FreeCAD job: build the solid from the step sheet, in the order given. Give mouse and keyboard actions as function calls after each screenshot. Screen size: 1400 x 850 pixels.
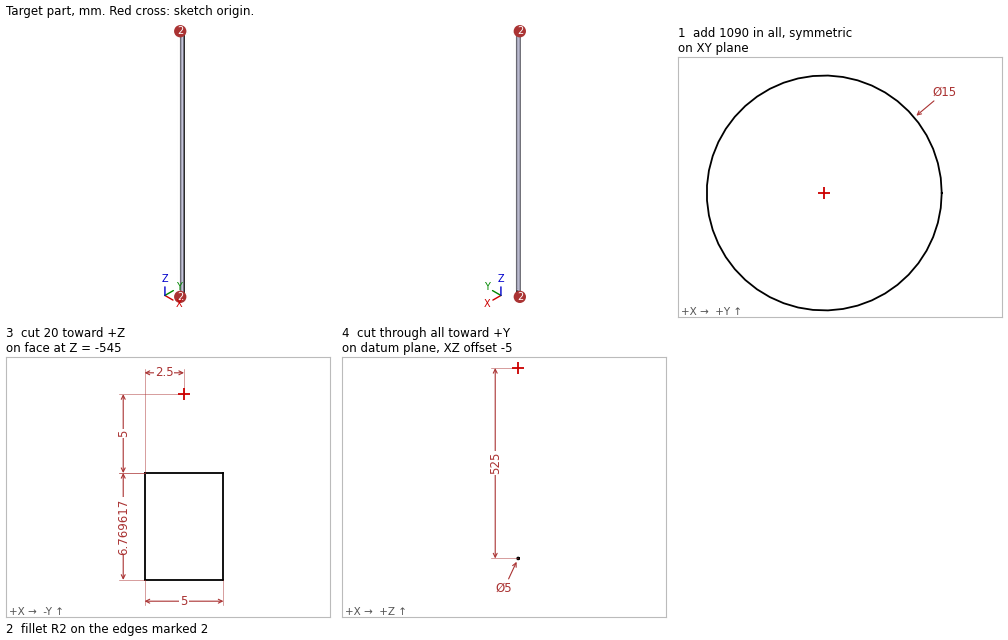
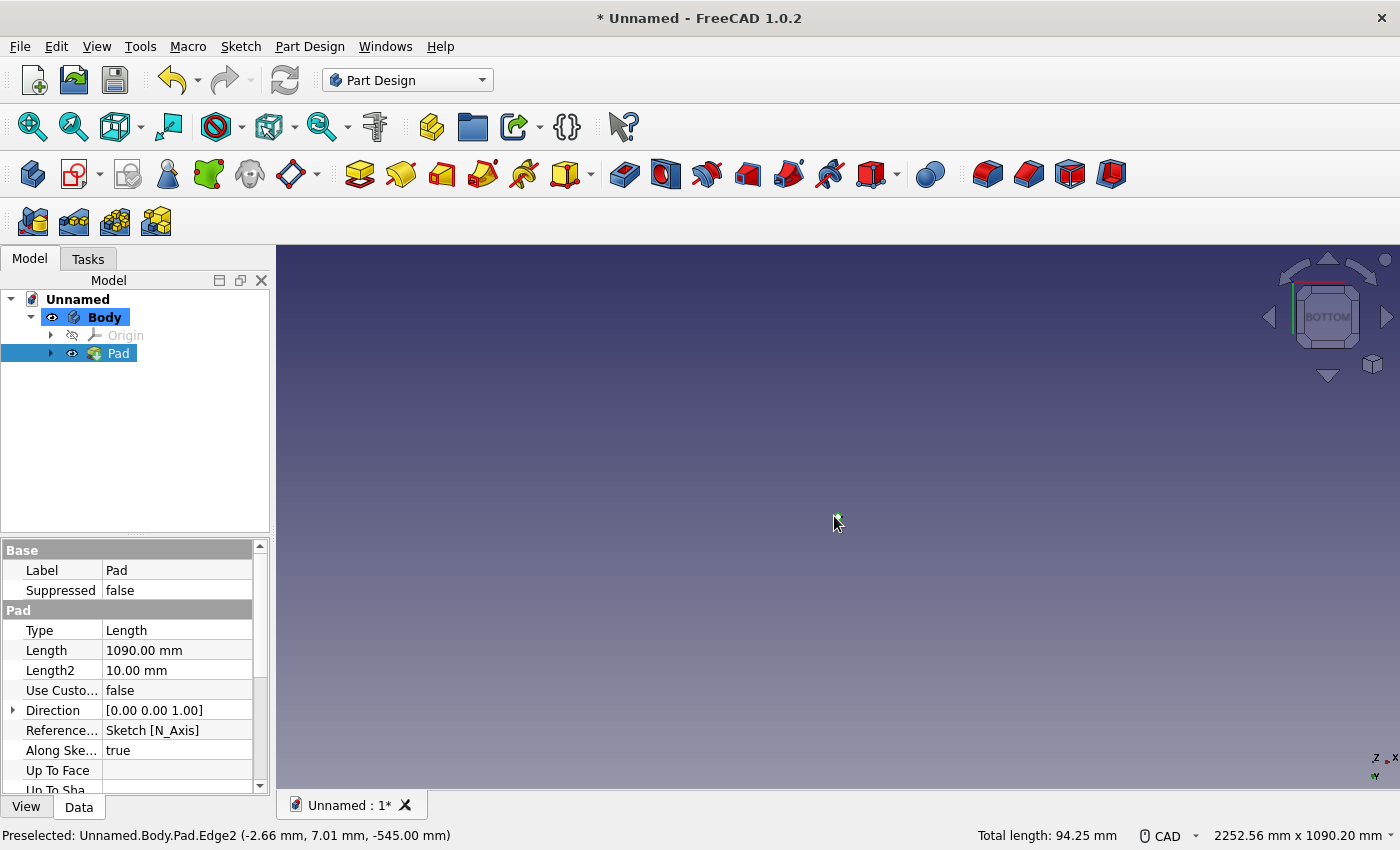
click(988, 174)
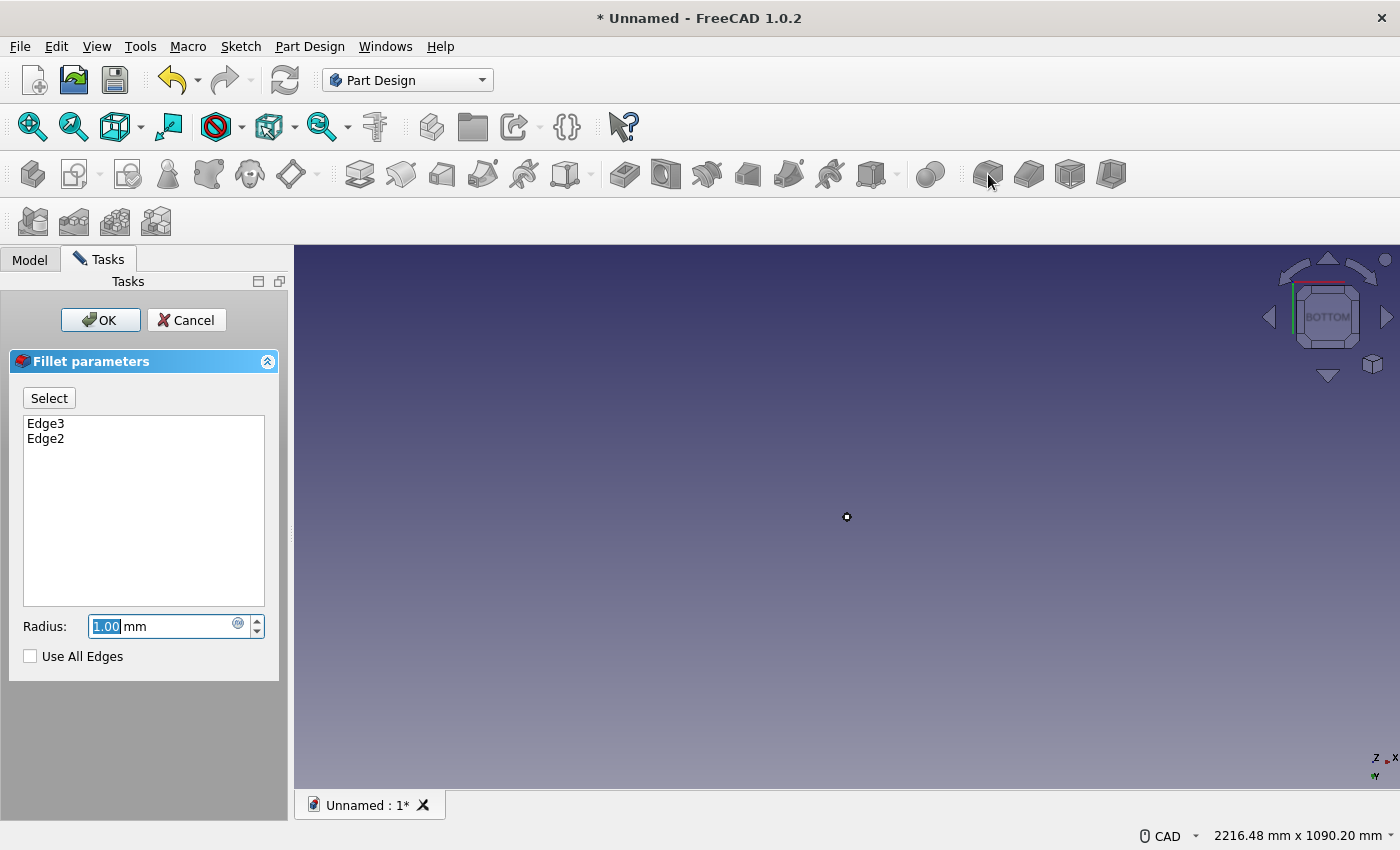
text(2)
key(Tab)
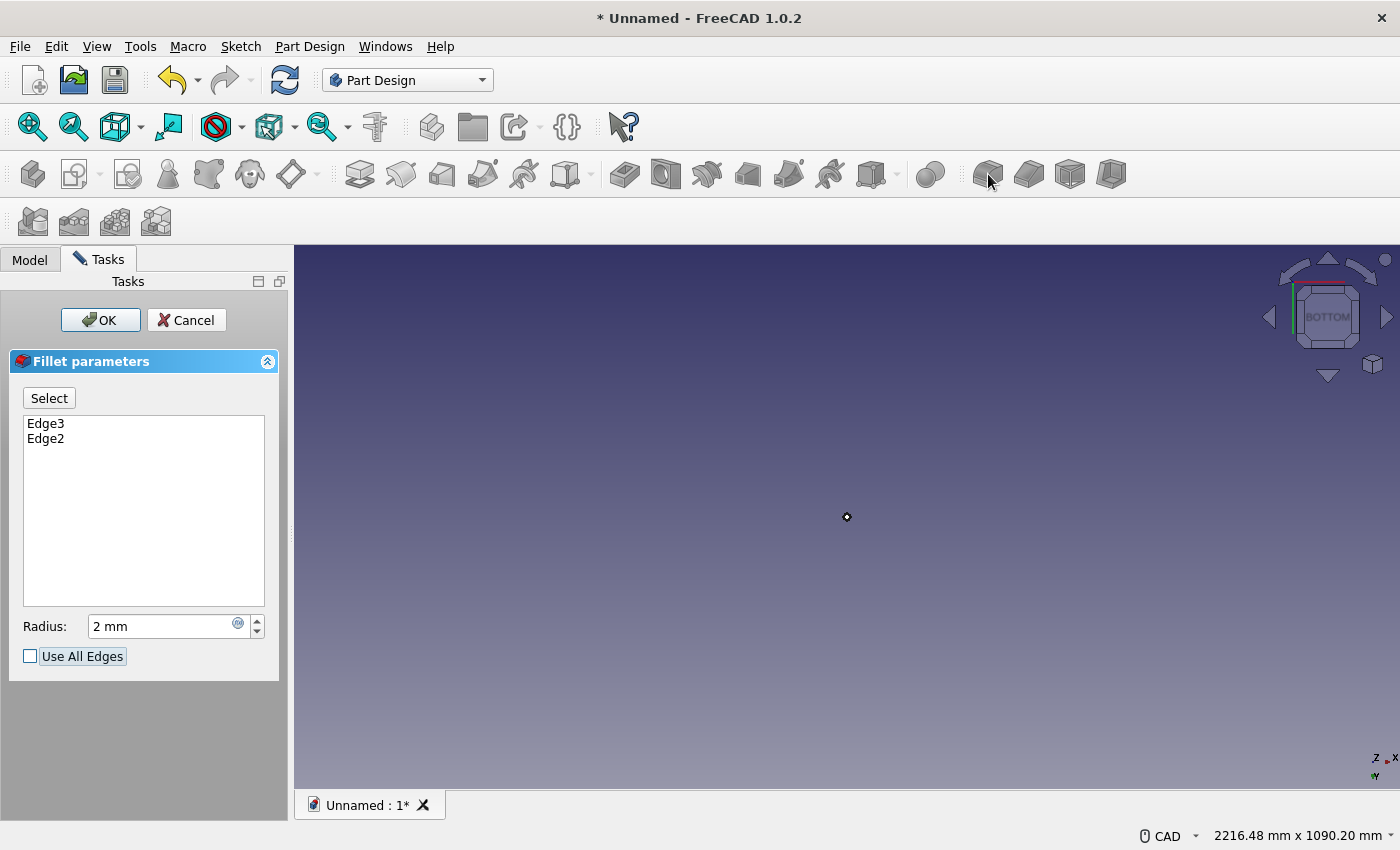
click(101, 320)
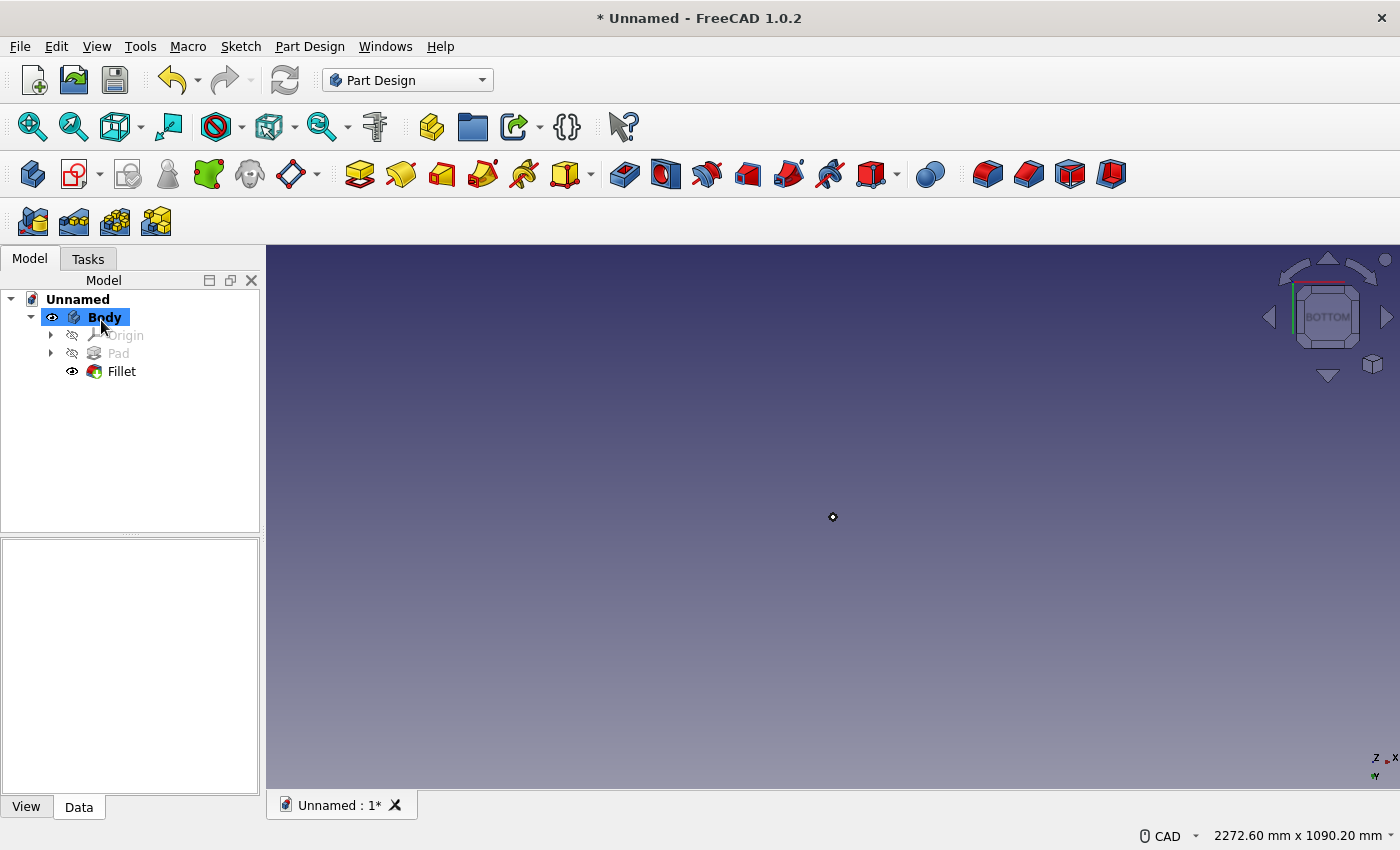
click(33, 128)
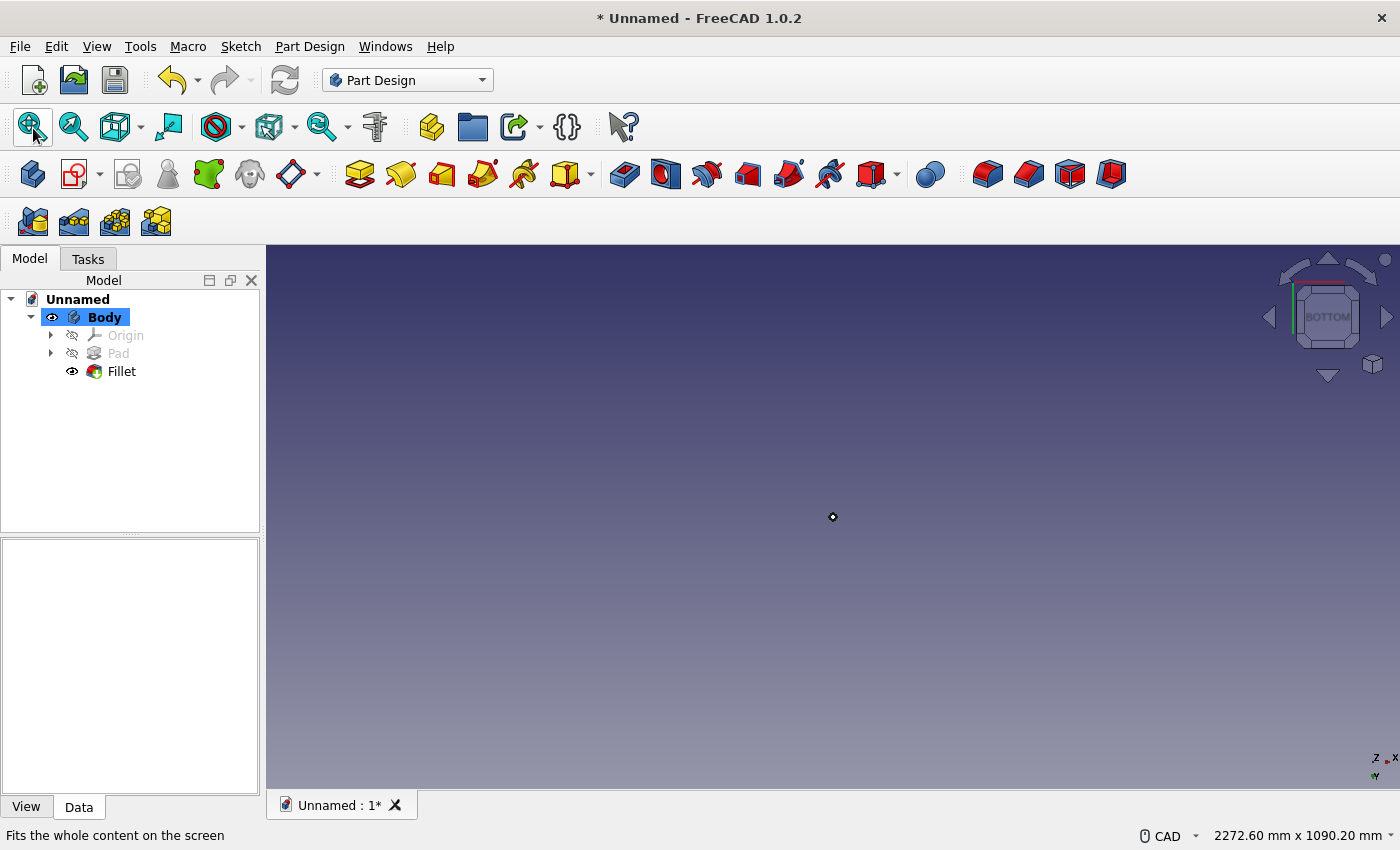
scroll(833, 516, up, 8)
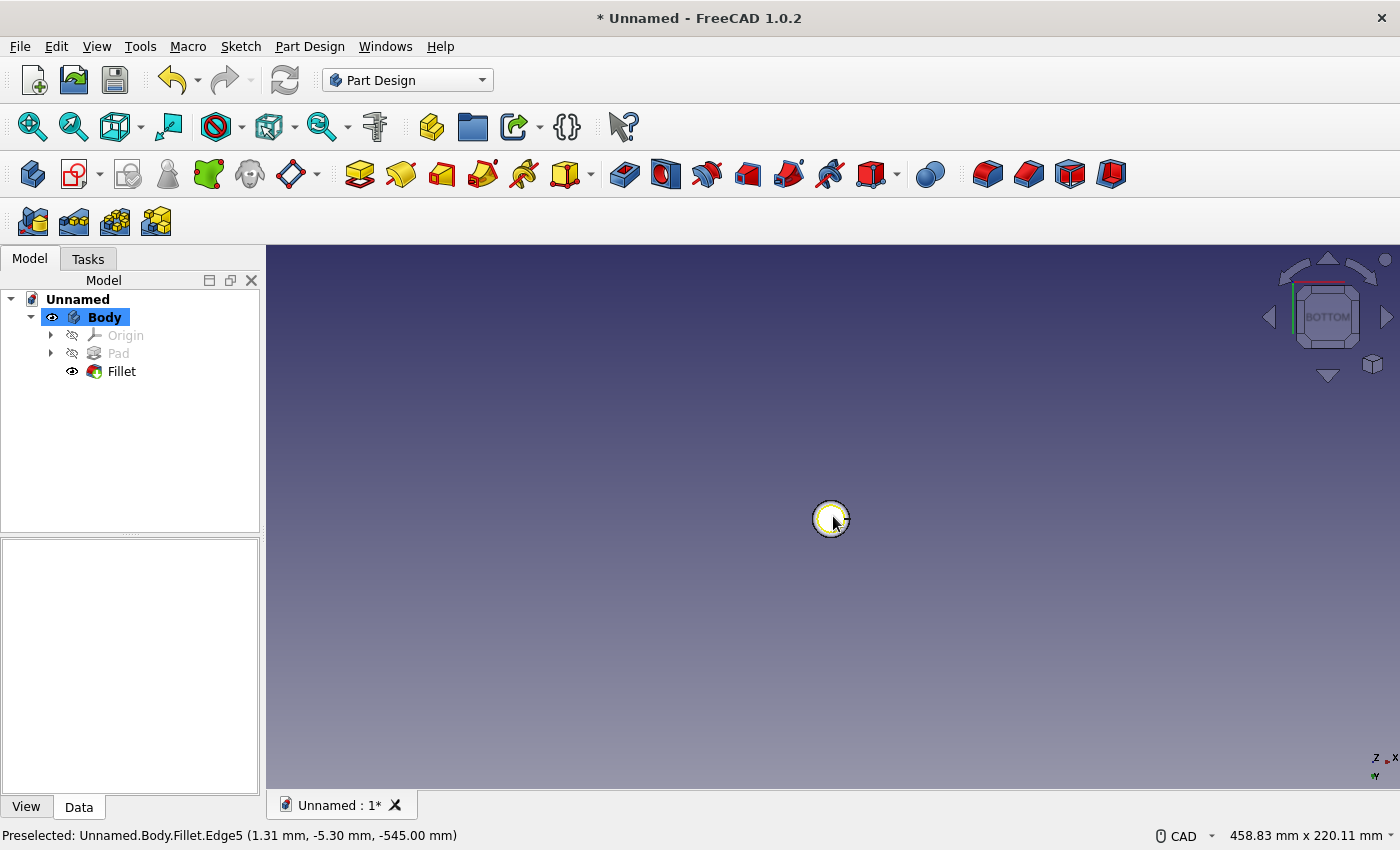
click(831, 518)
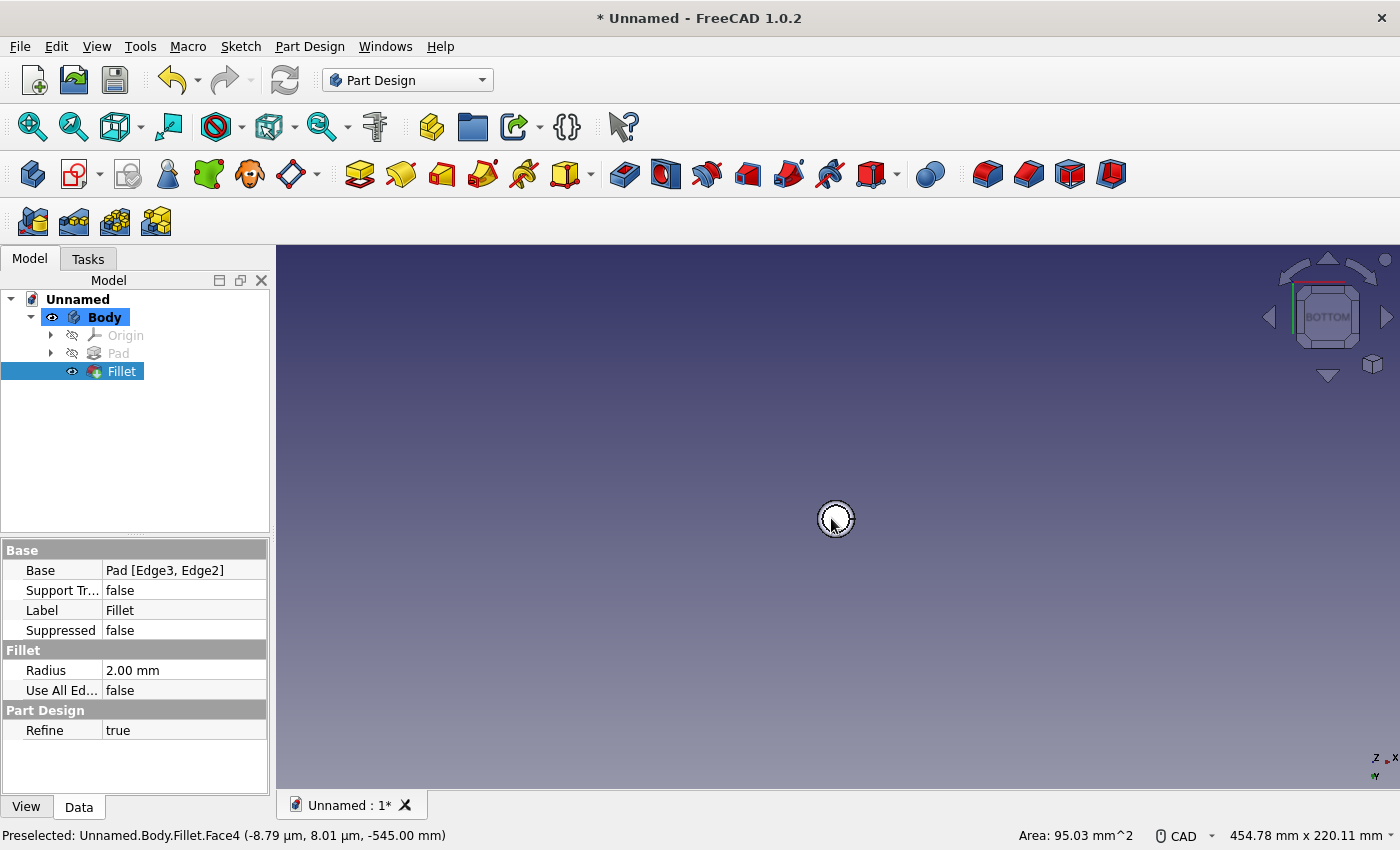
click(74, 174)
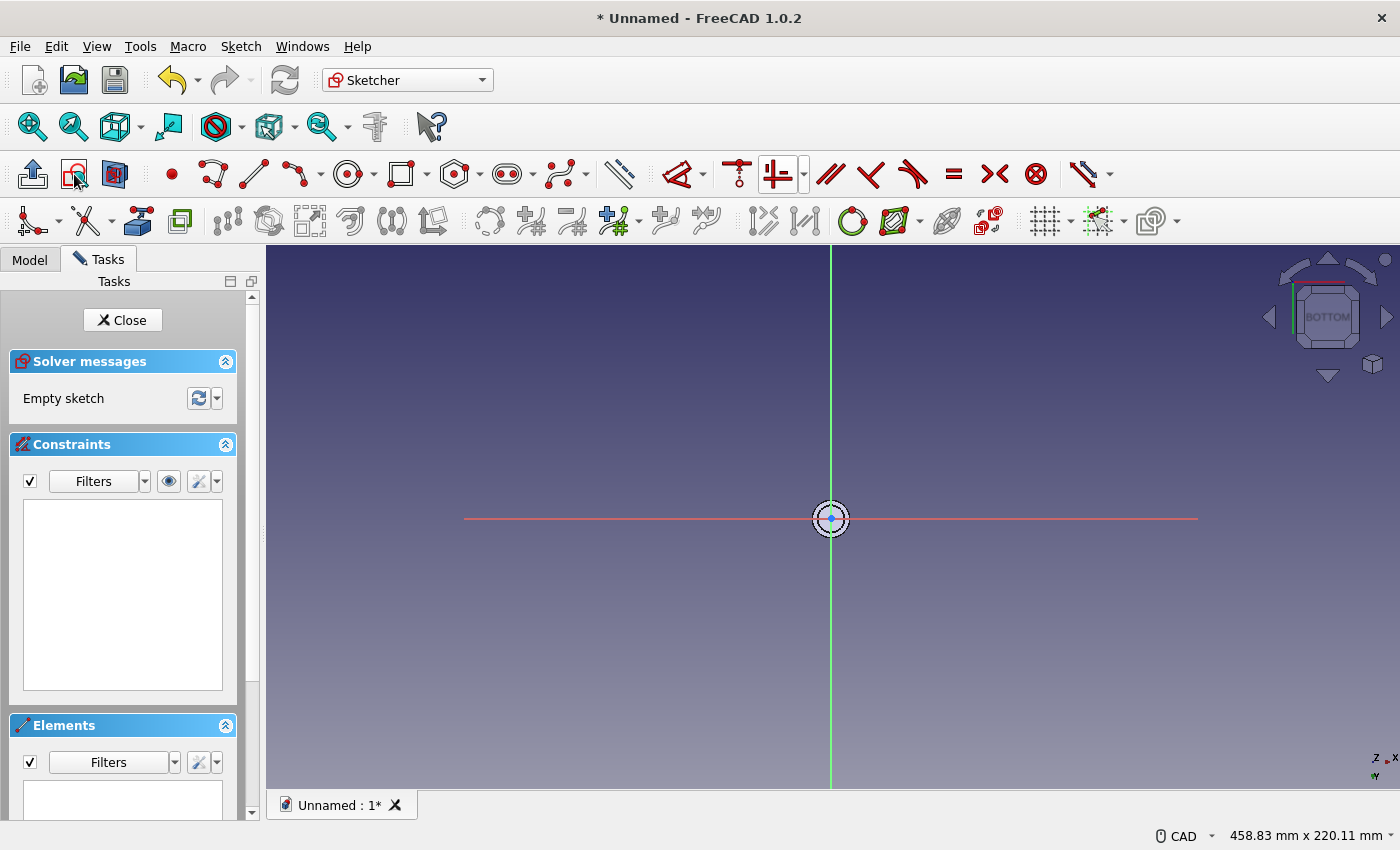
scroll(838, 535, up, 12)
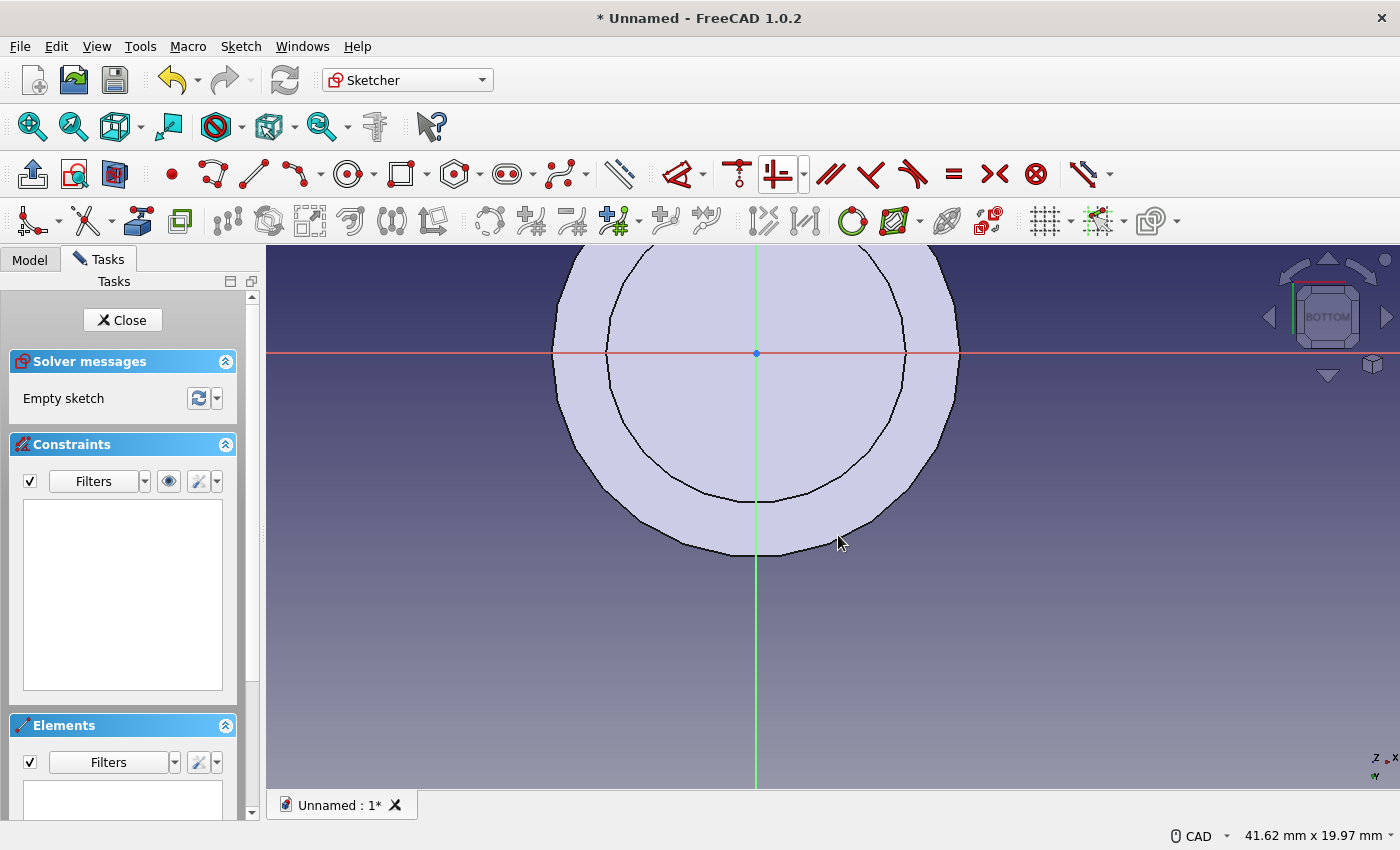
click(400, 174)